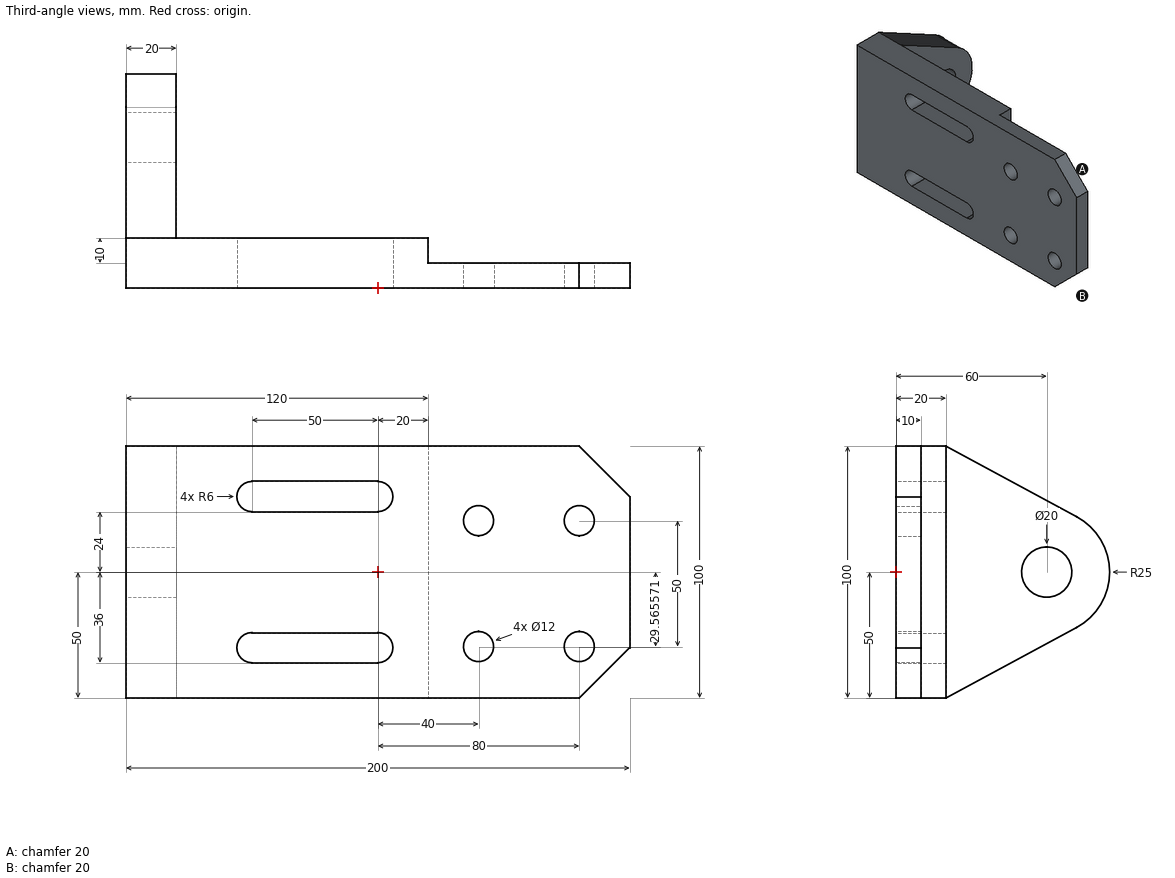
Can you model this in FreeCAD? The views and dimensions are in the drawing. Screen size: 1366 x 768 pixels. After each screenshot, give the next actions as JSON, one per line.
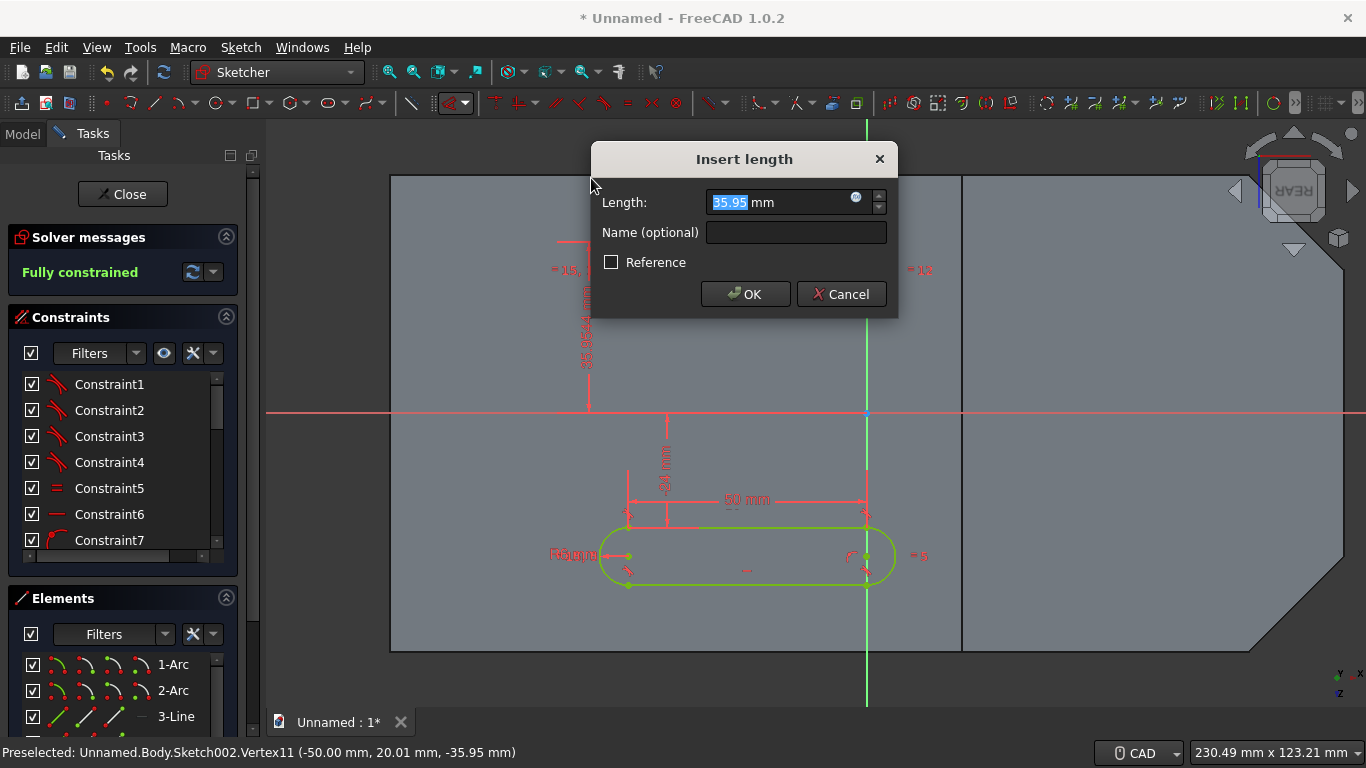
{"action": "type", "text": "36"}
{"action": "key", "text": "Return"}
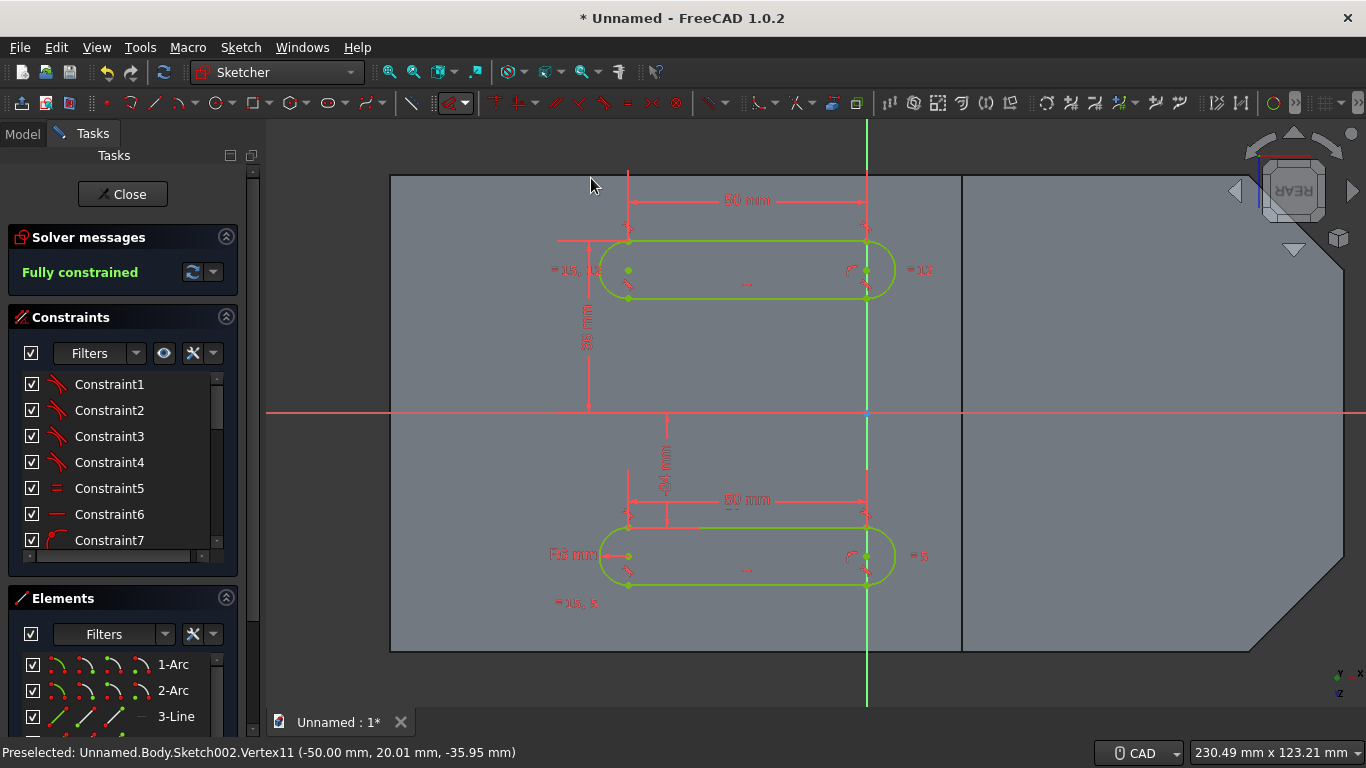
{"action": "left_click", "coordinate": [123, 194]}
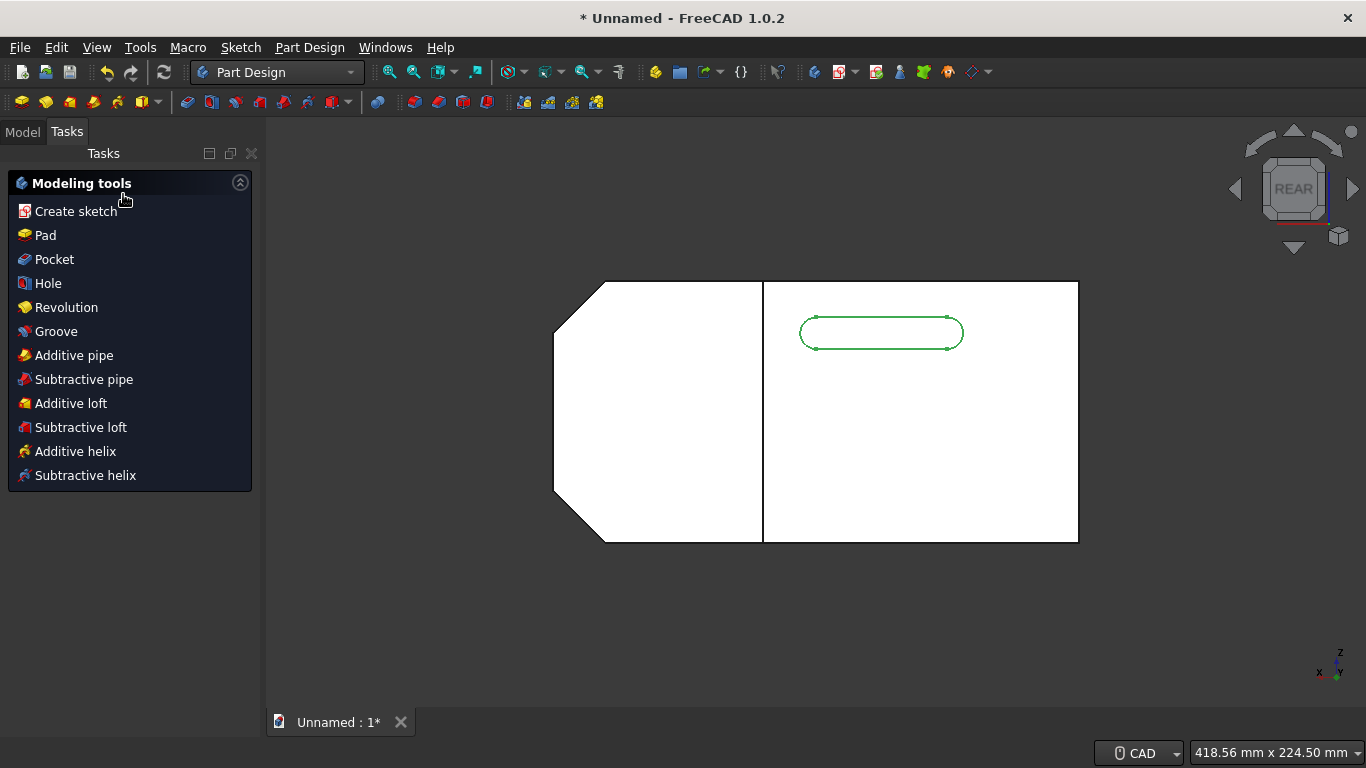
{"action": "left_click", "coordinate": [188, 102]}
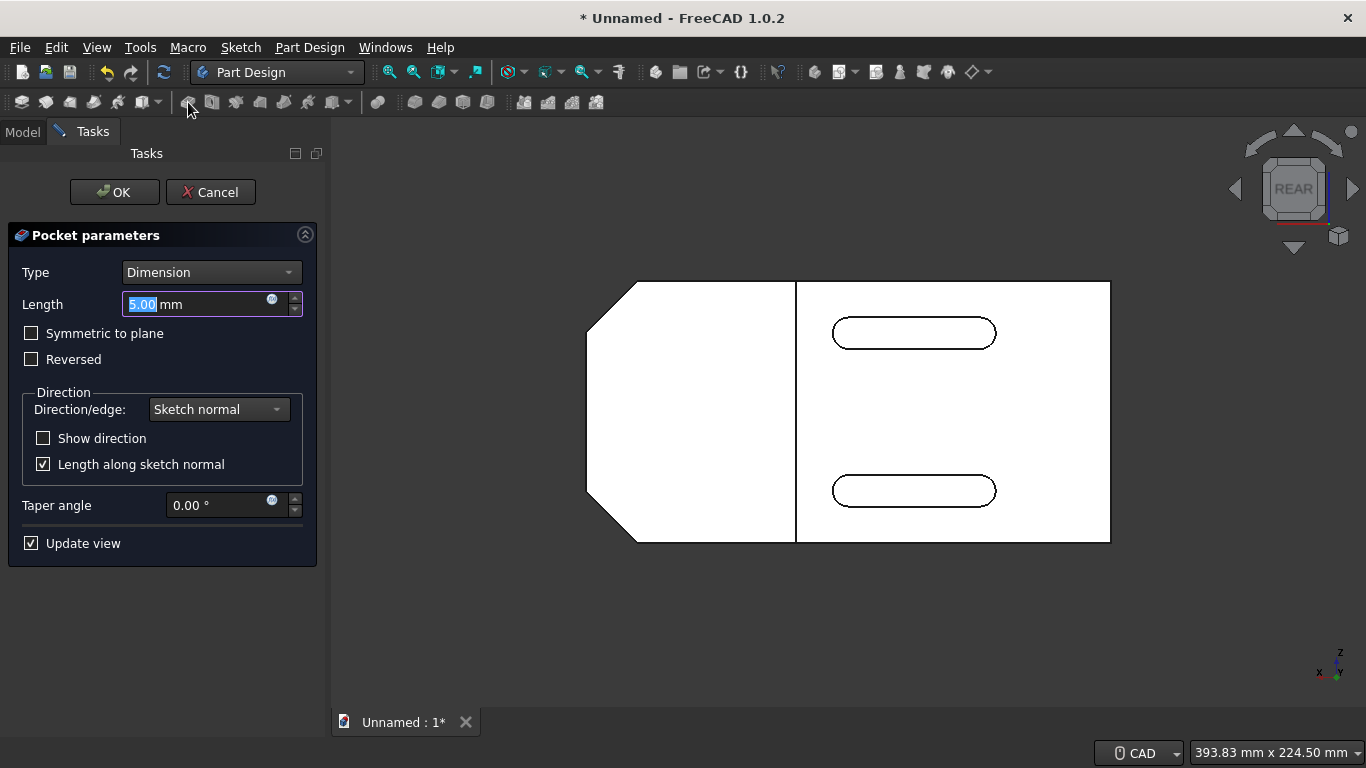
{"action": "type", "text": "20"}
{"action": "key", "text": "Tab"}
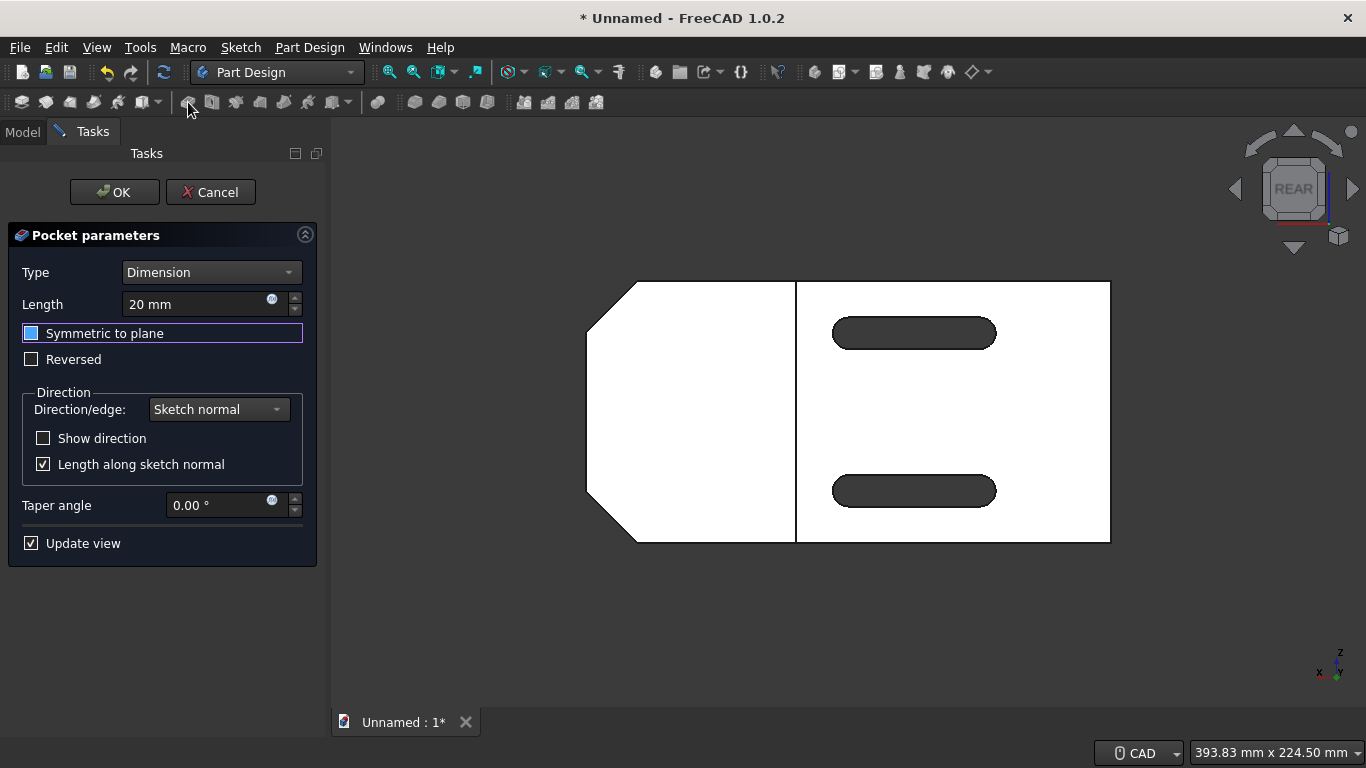
{"action": "left_click", "coordinate": [115, 192]}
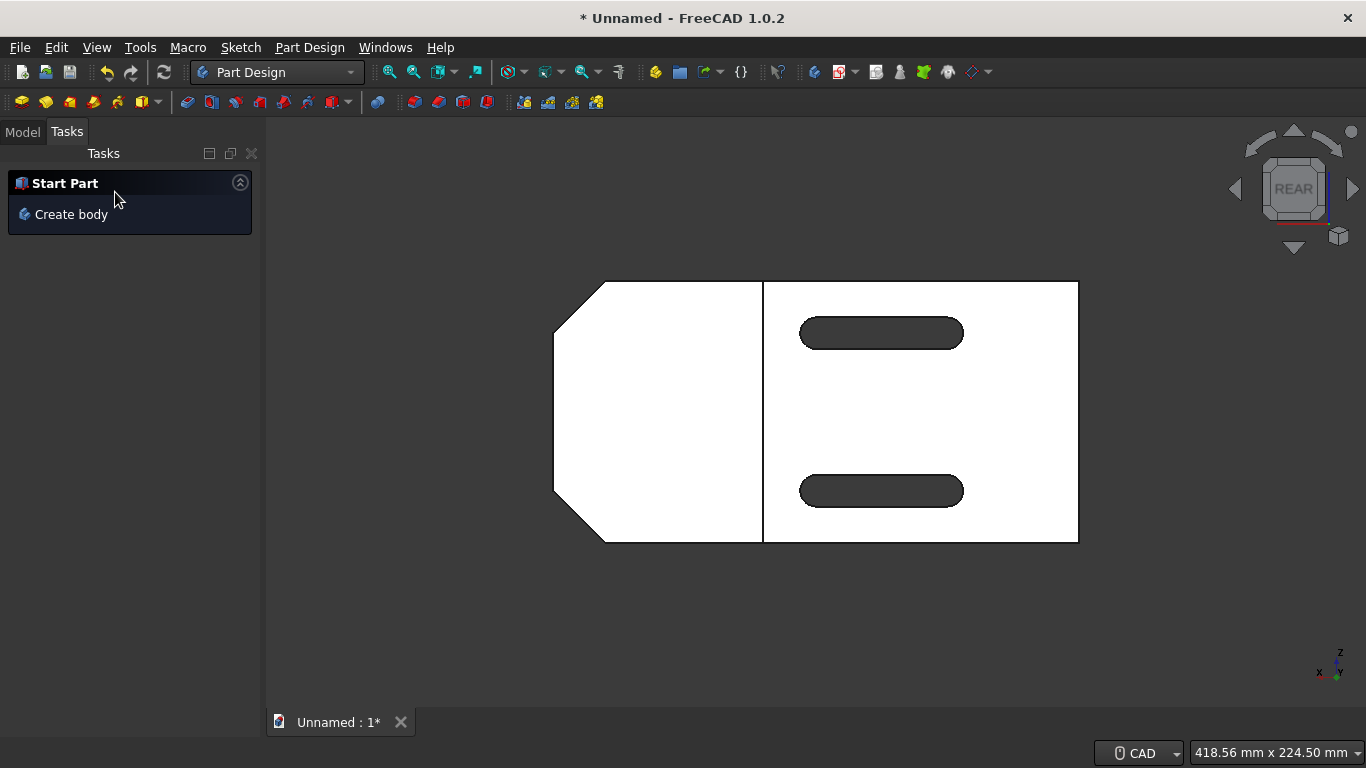
{"action": "key", "text": "6"}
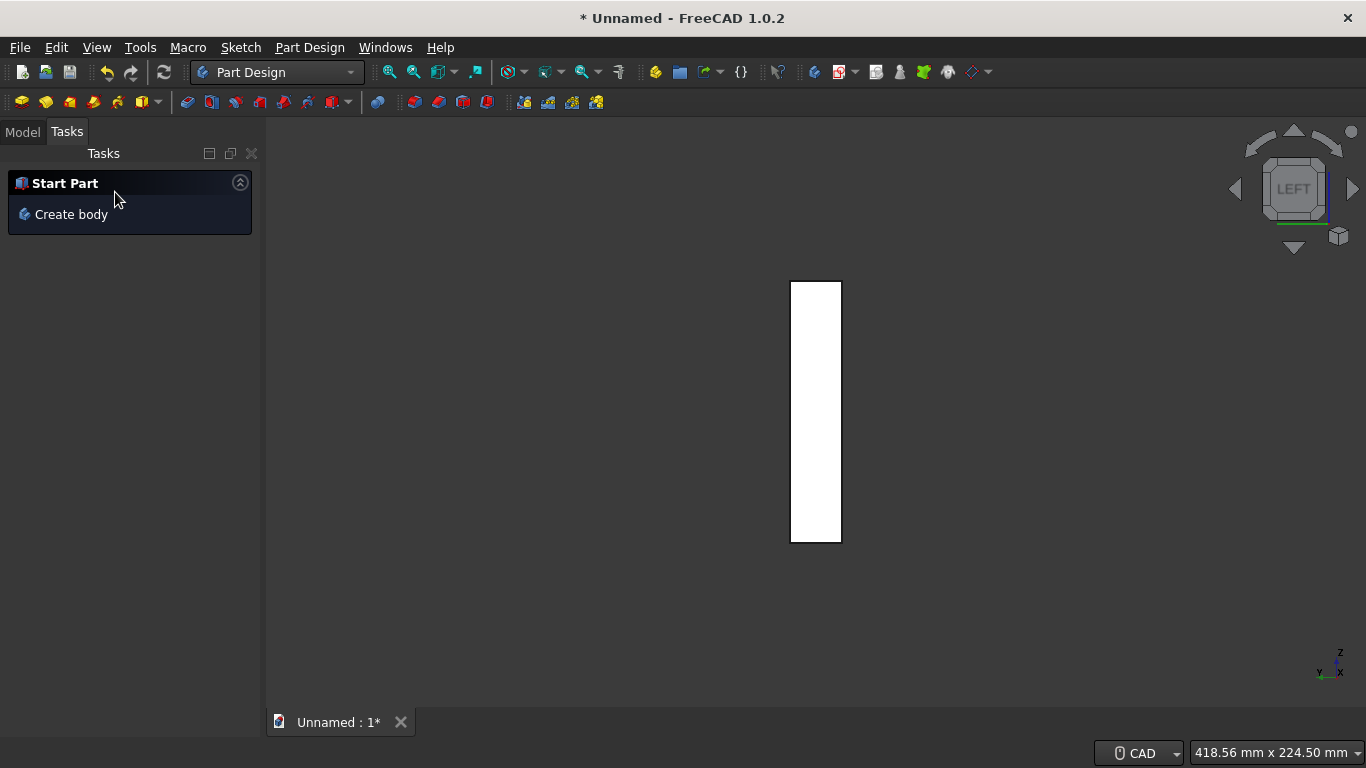
{"action": "left_click", "coordinate": [390, 72]}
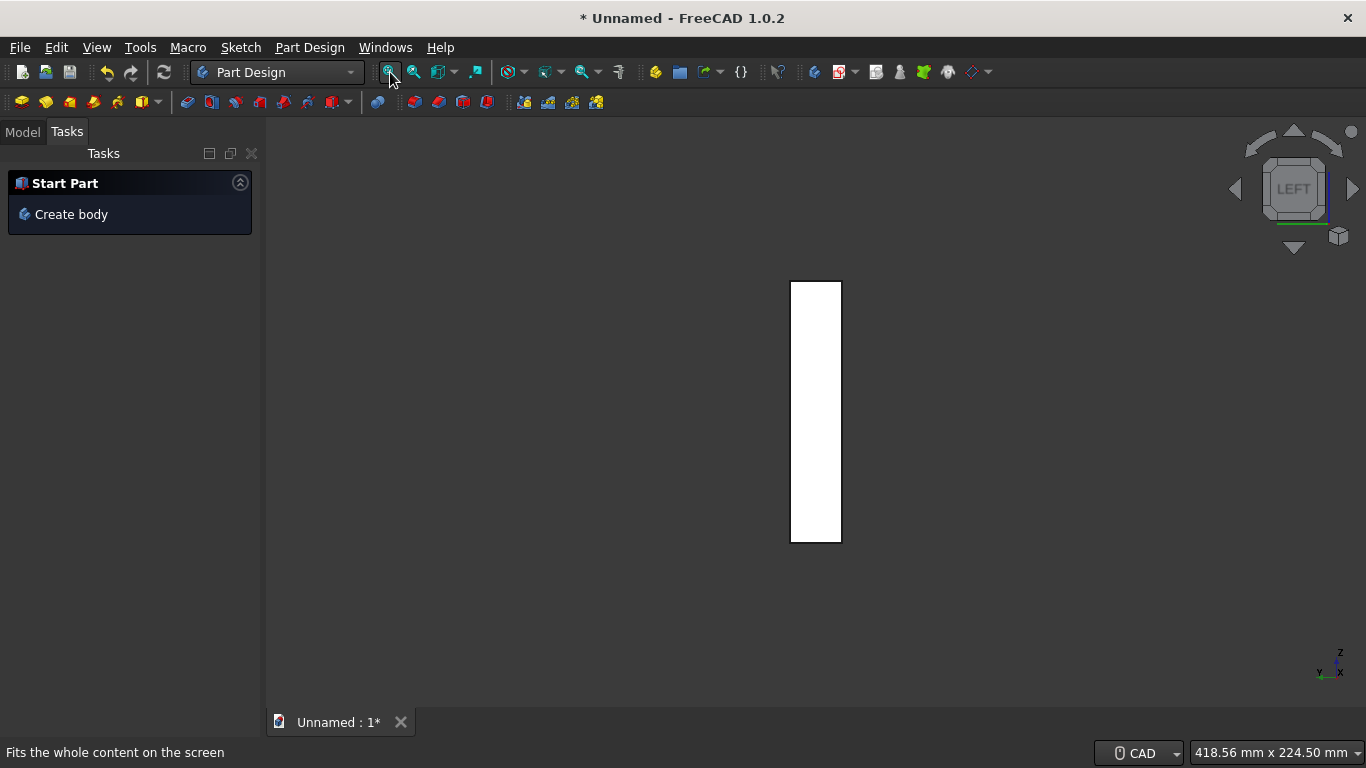
{"action": "left_click", "coordinate": [816, 486]}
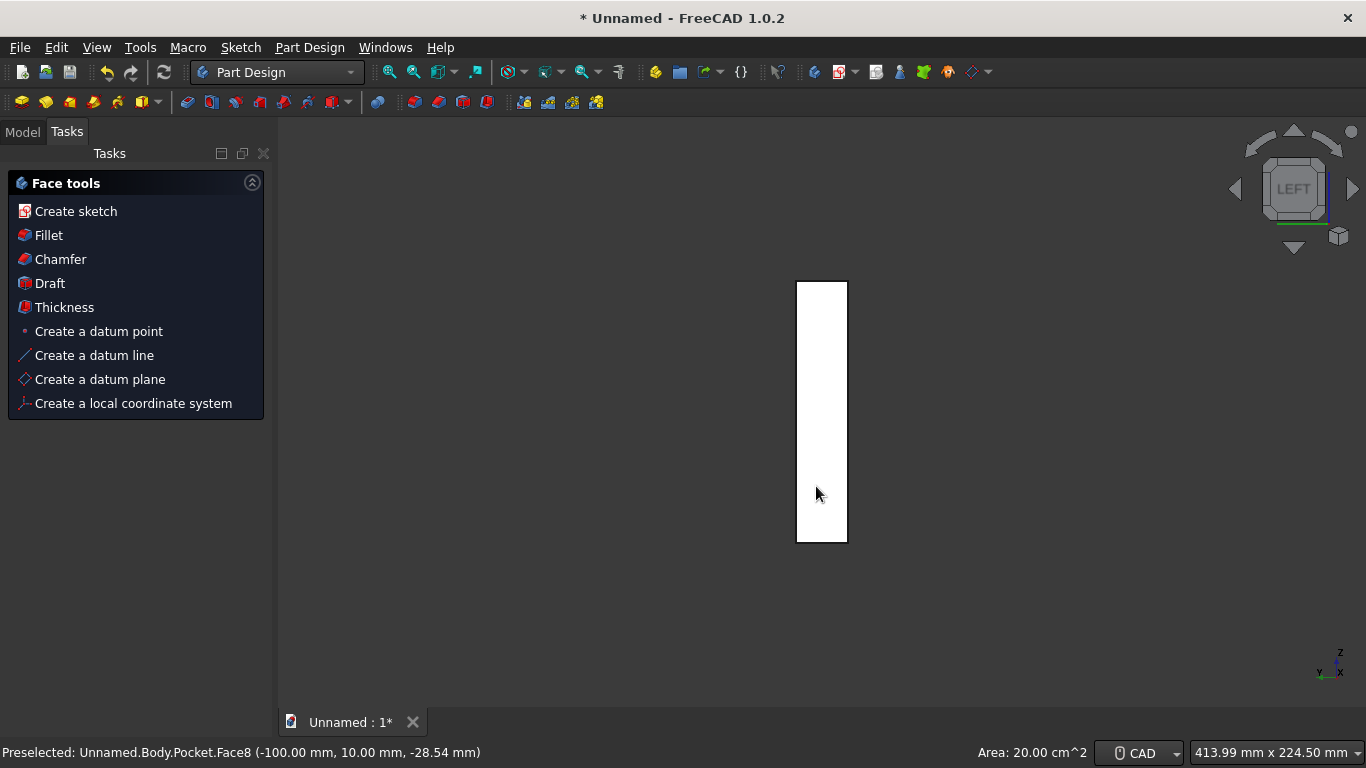
{"action": "left_click", "coordinate": [840, 72]}